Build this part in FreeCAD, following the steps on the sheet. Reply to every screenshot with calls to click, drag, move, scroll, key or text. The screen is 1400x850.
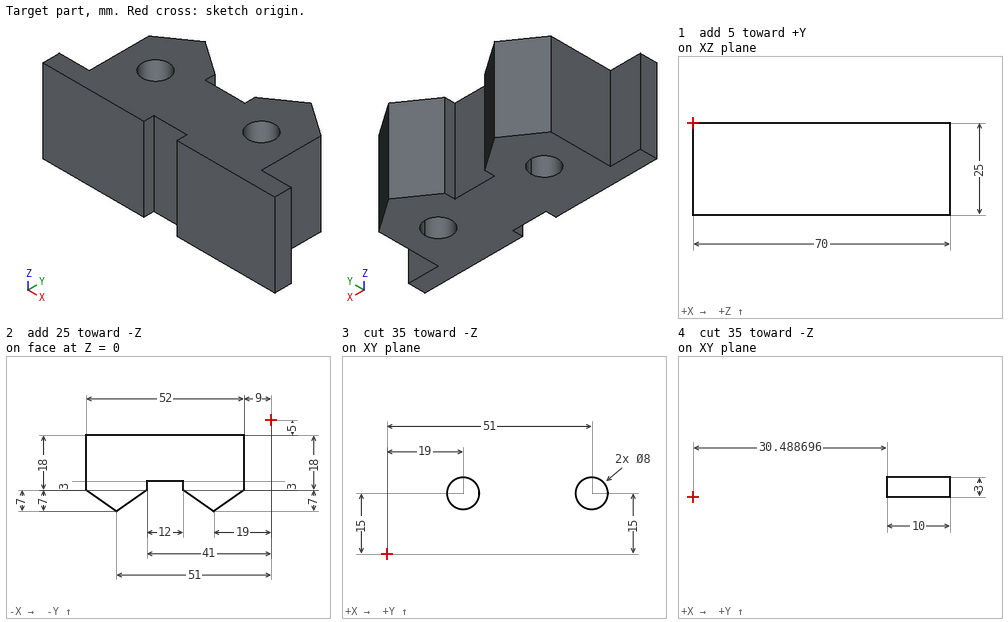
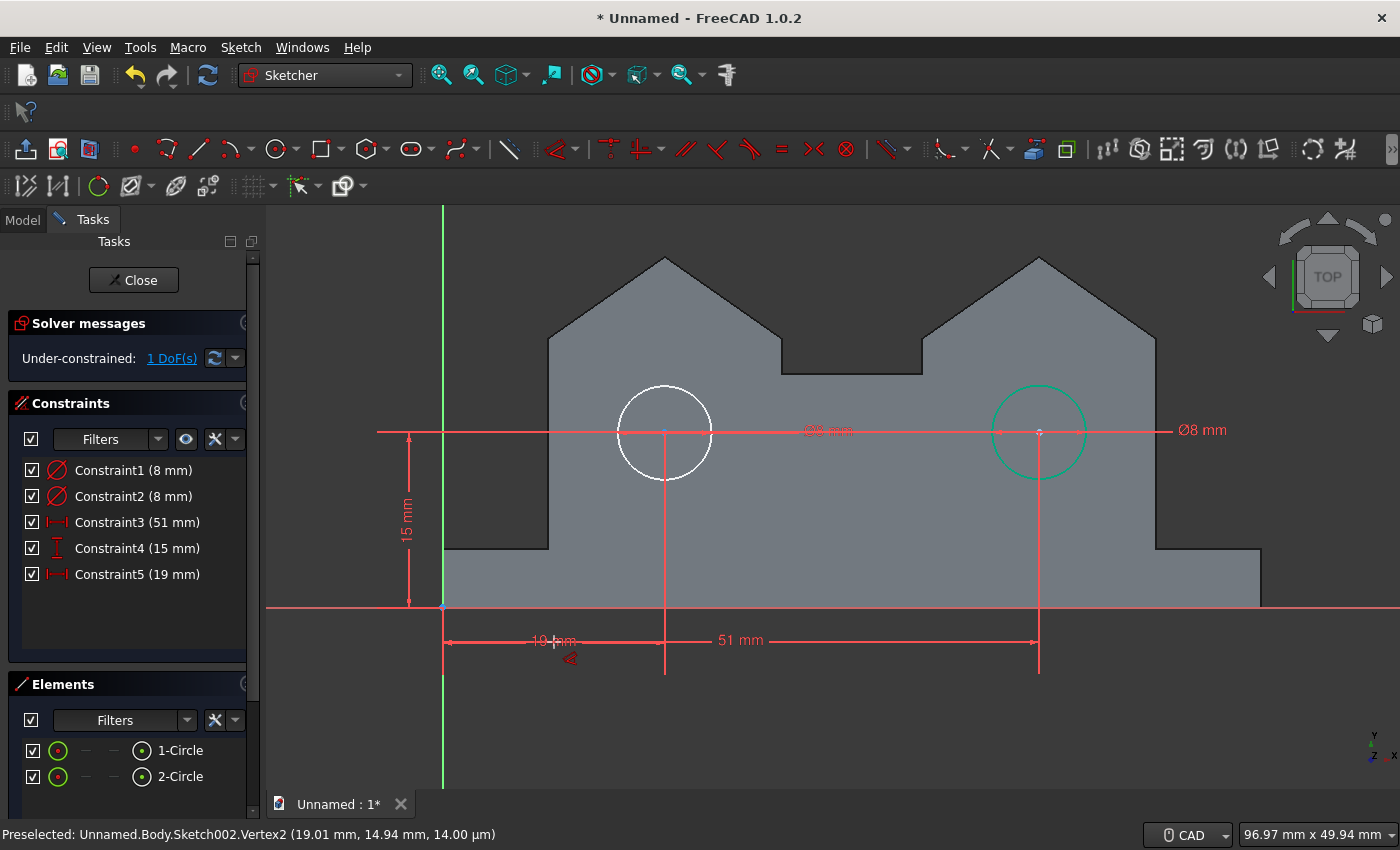
click(665, 433)
click(409, 480)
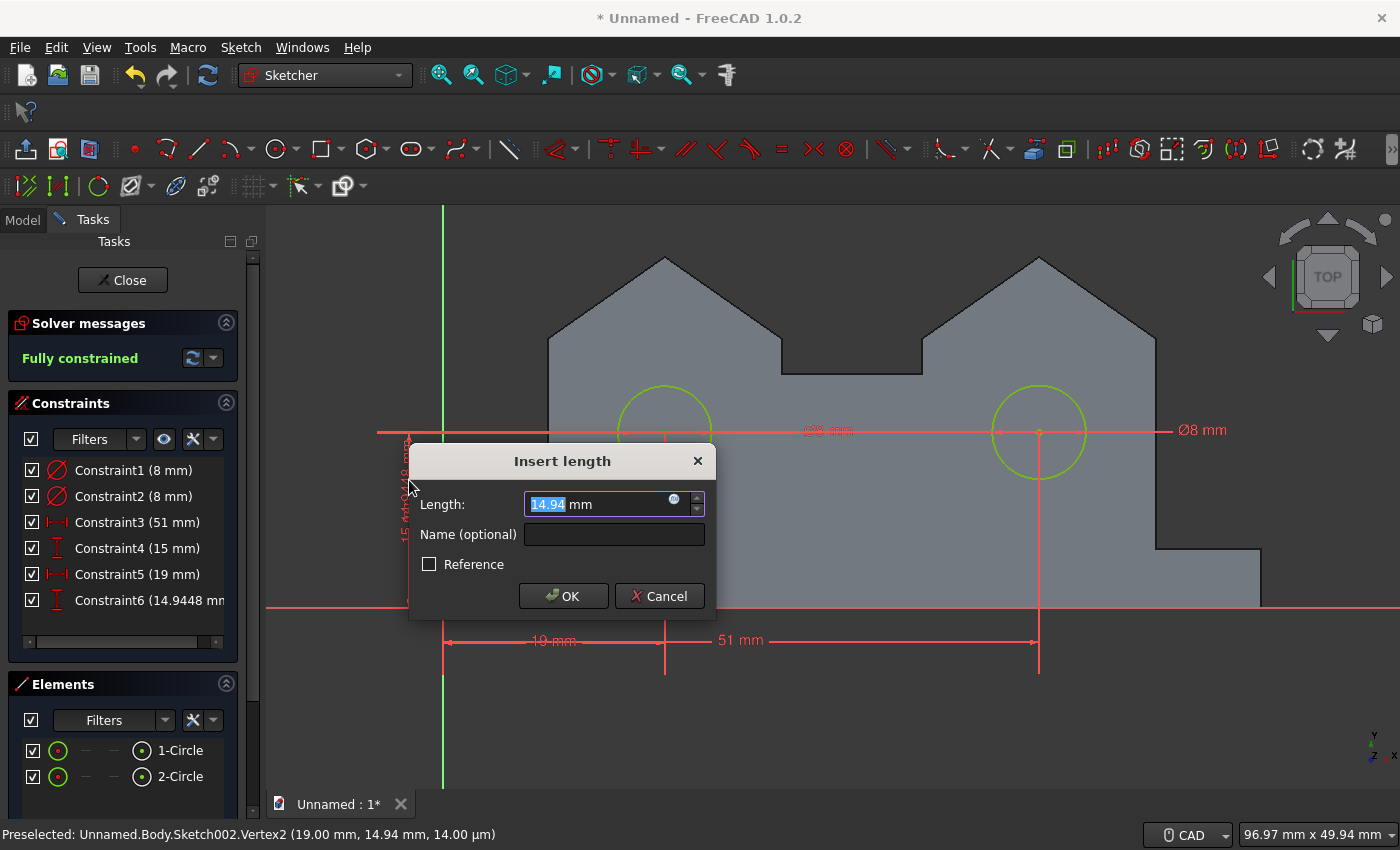
text(15)
key(Return)
key(Escape)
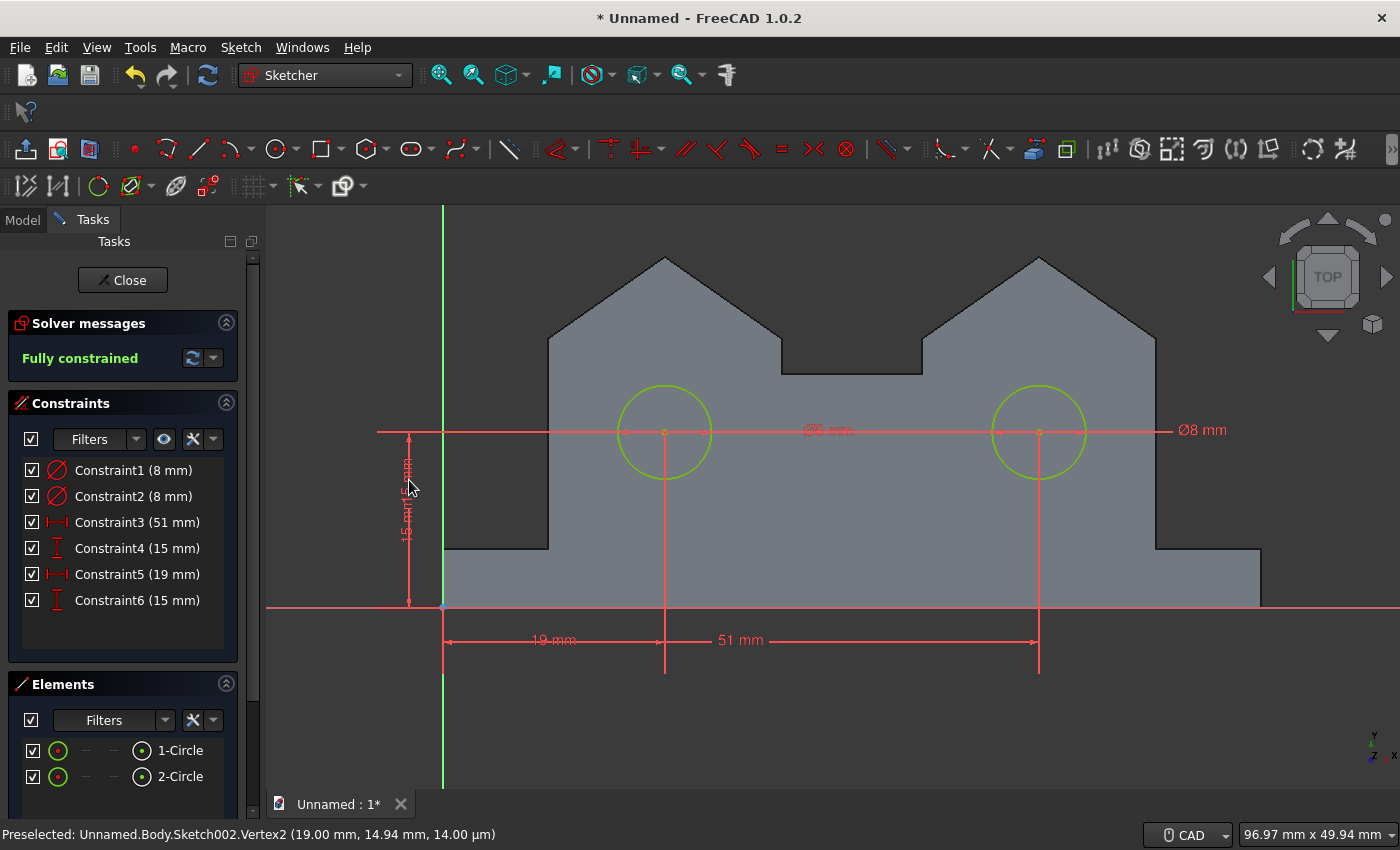
click(123, 280)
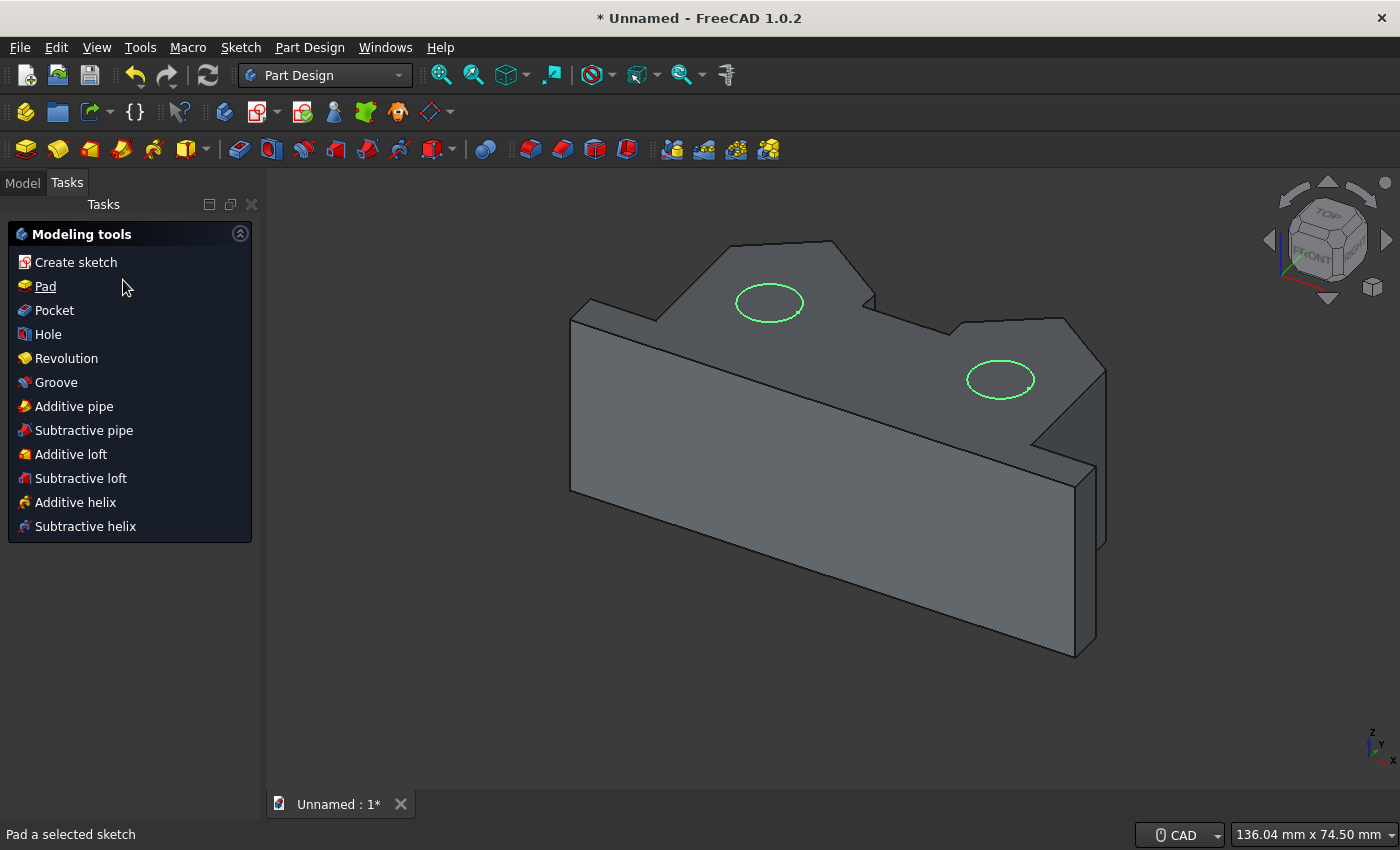
click(240, 150)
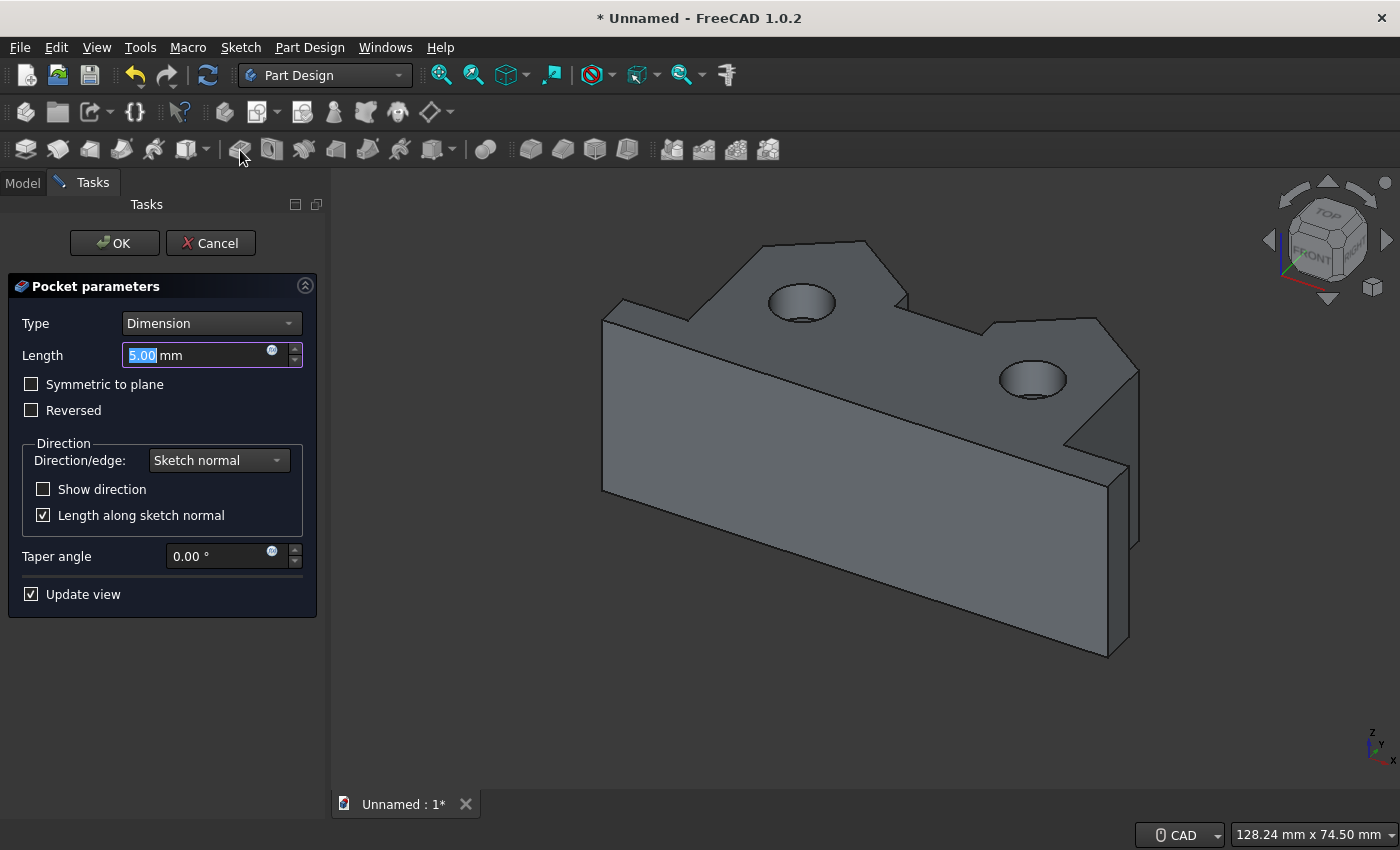
text(35)
key(Tab)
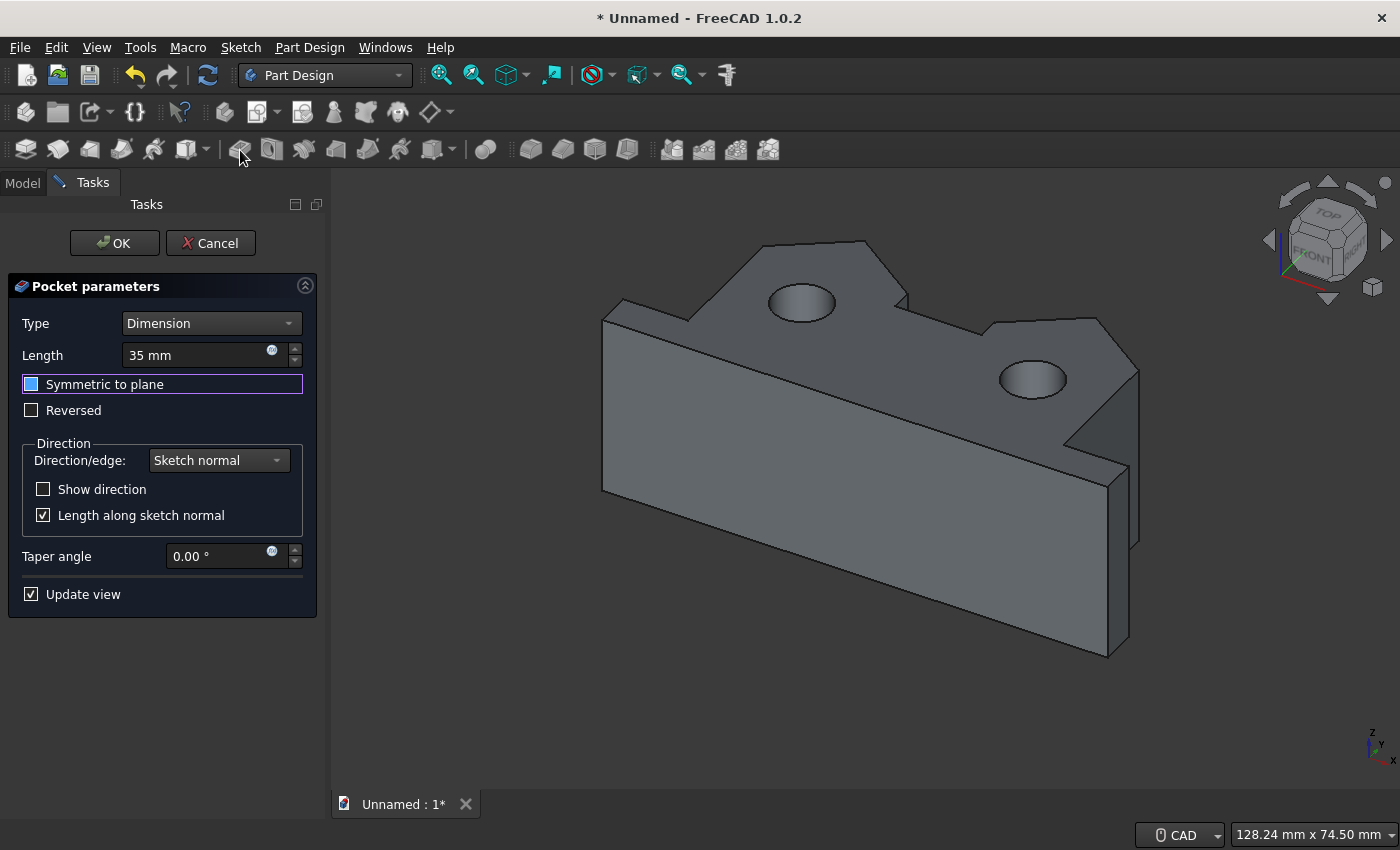
click(115, 243)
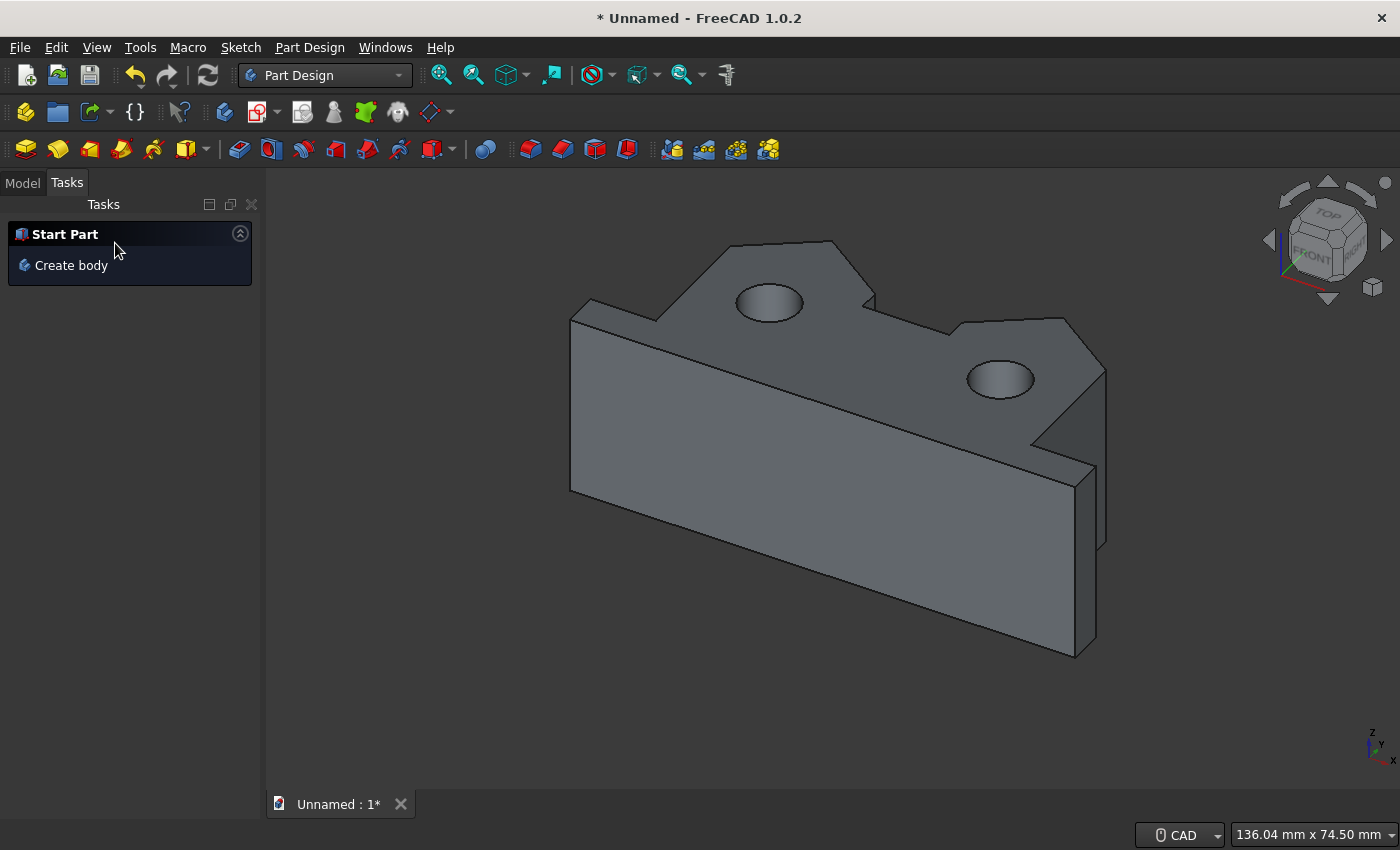
click(258, 112)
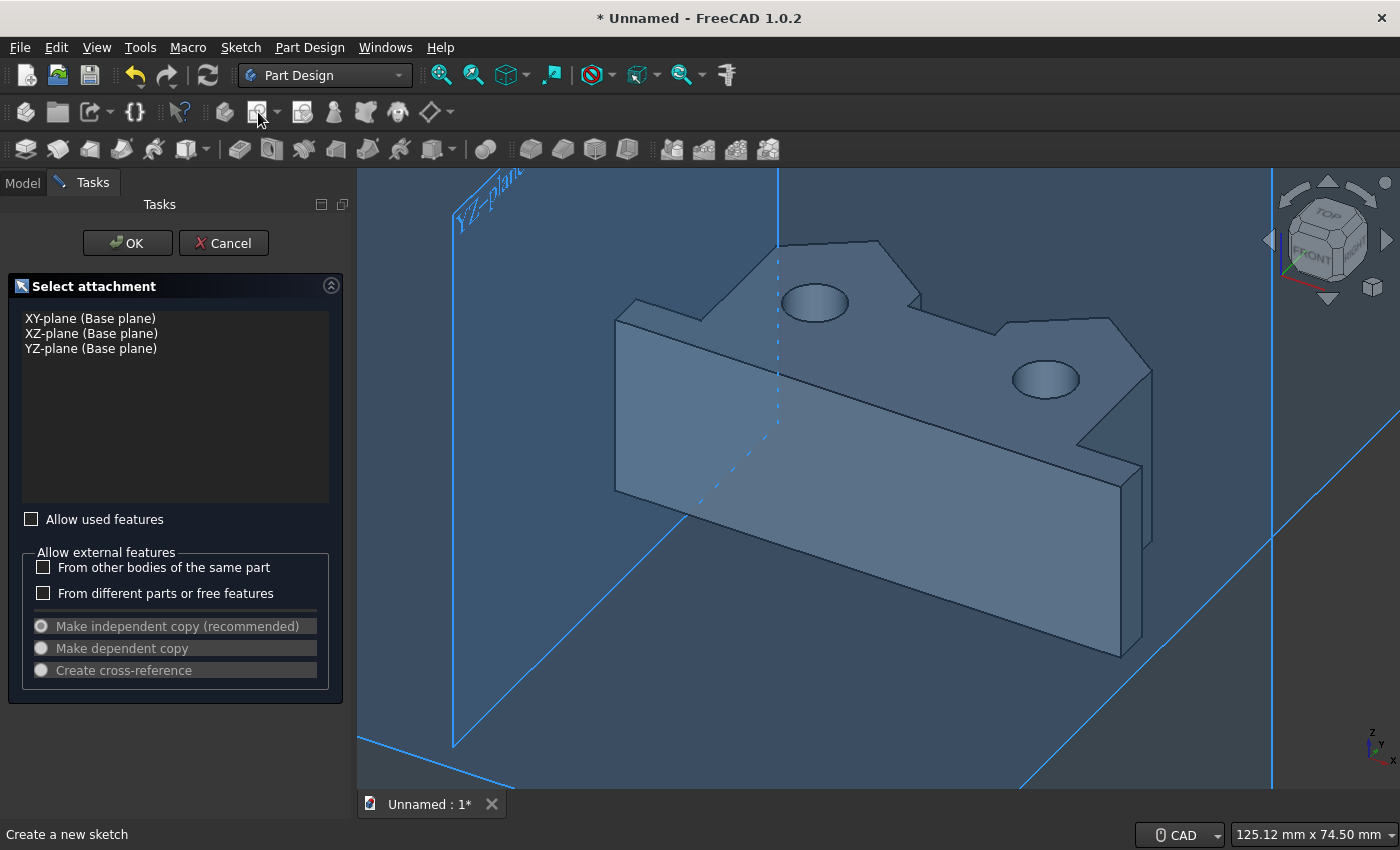
click(82, 318)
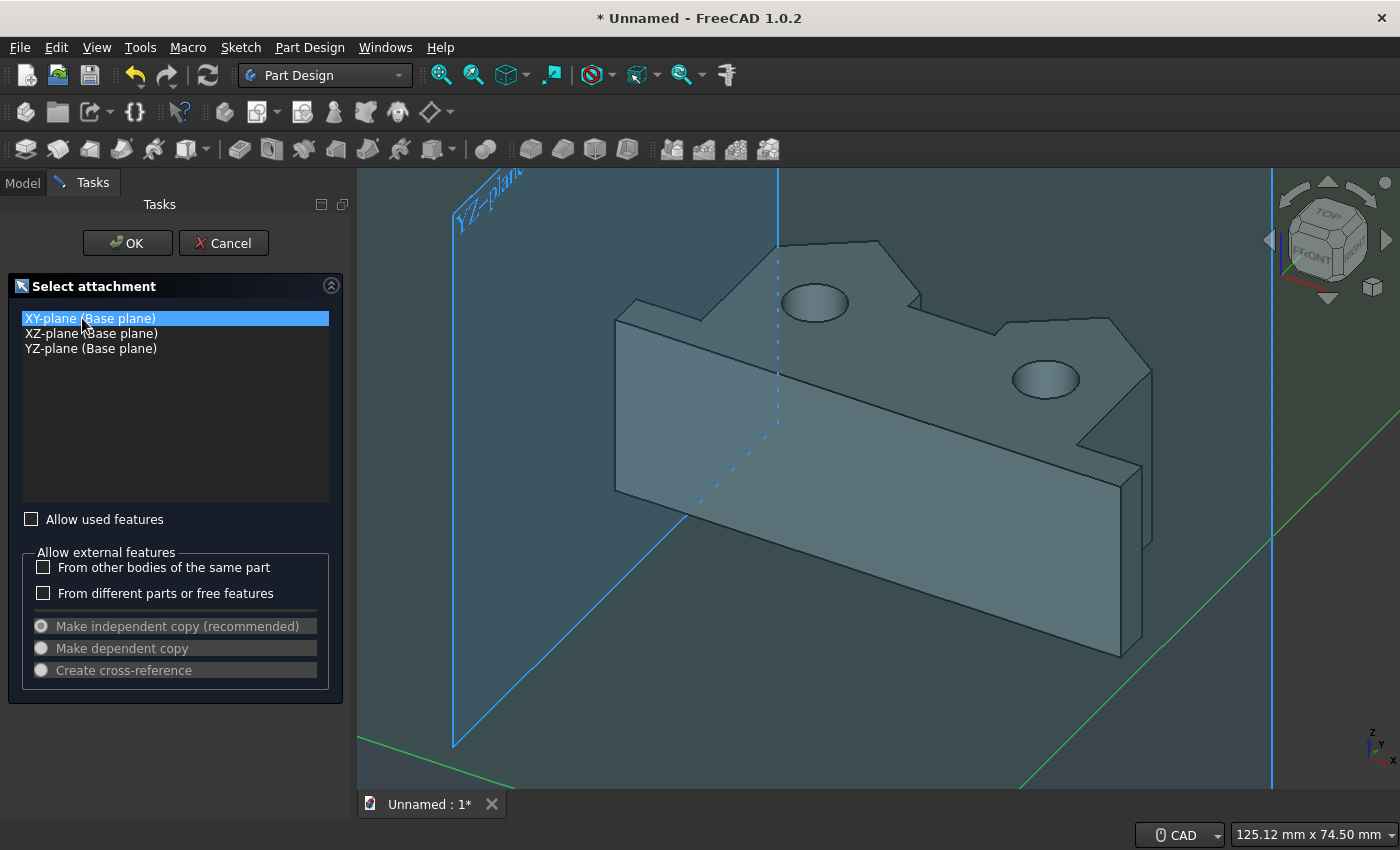
click(128, 243)